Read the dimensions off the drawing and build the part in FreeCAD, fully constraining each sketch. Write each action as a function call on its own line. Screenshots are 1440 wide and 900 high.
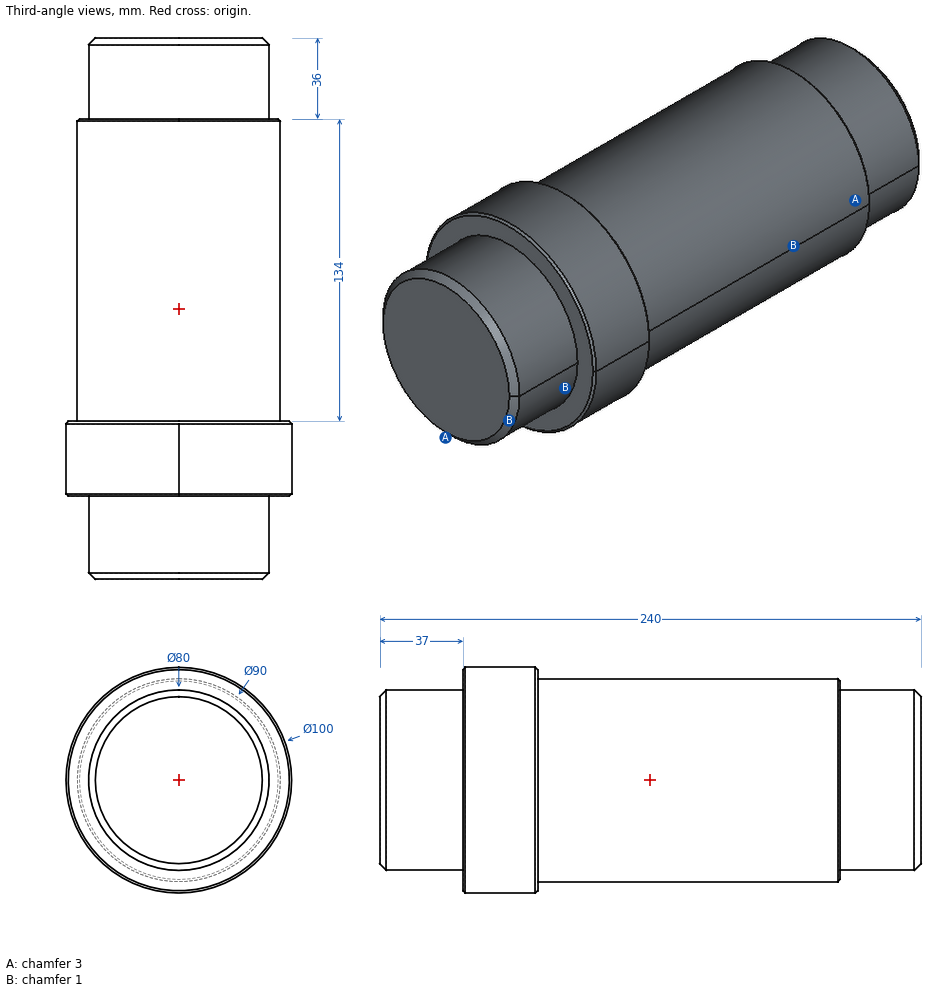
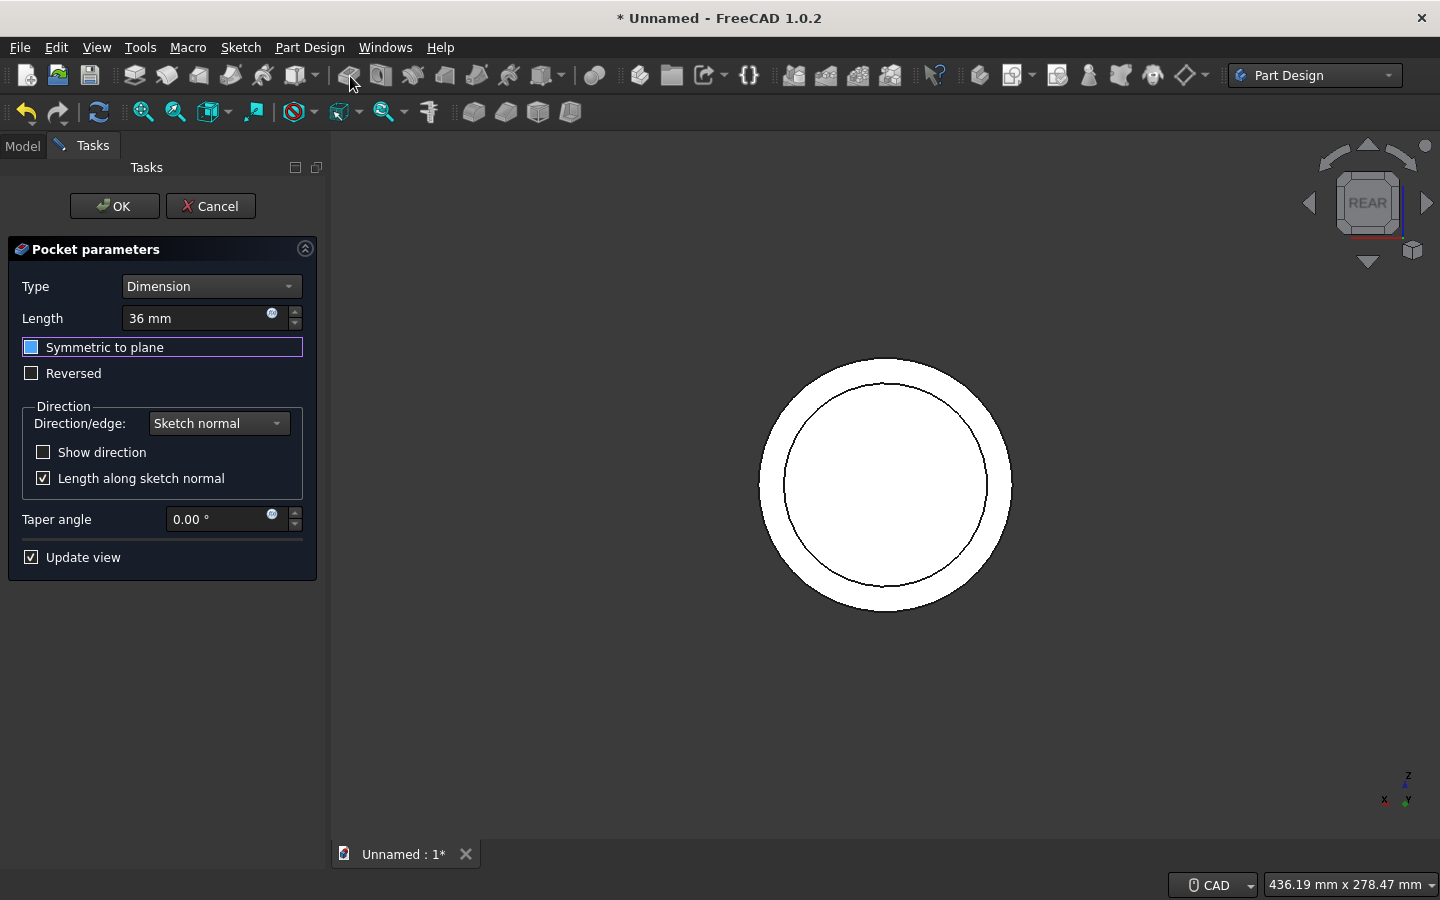
click(115, 206)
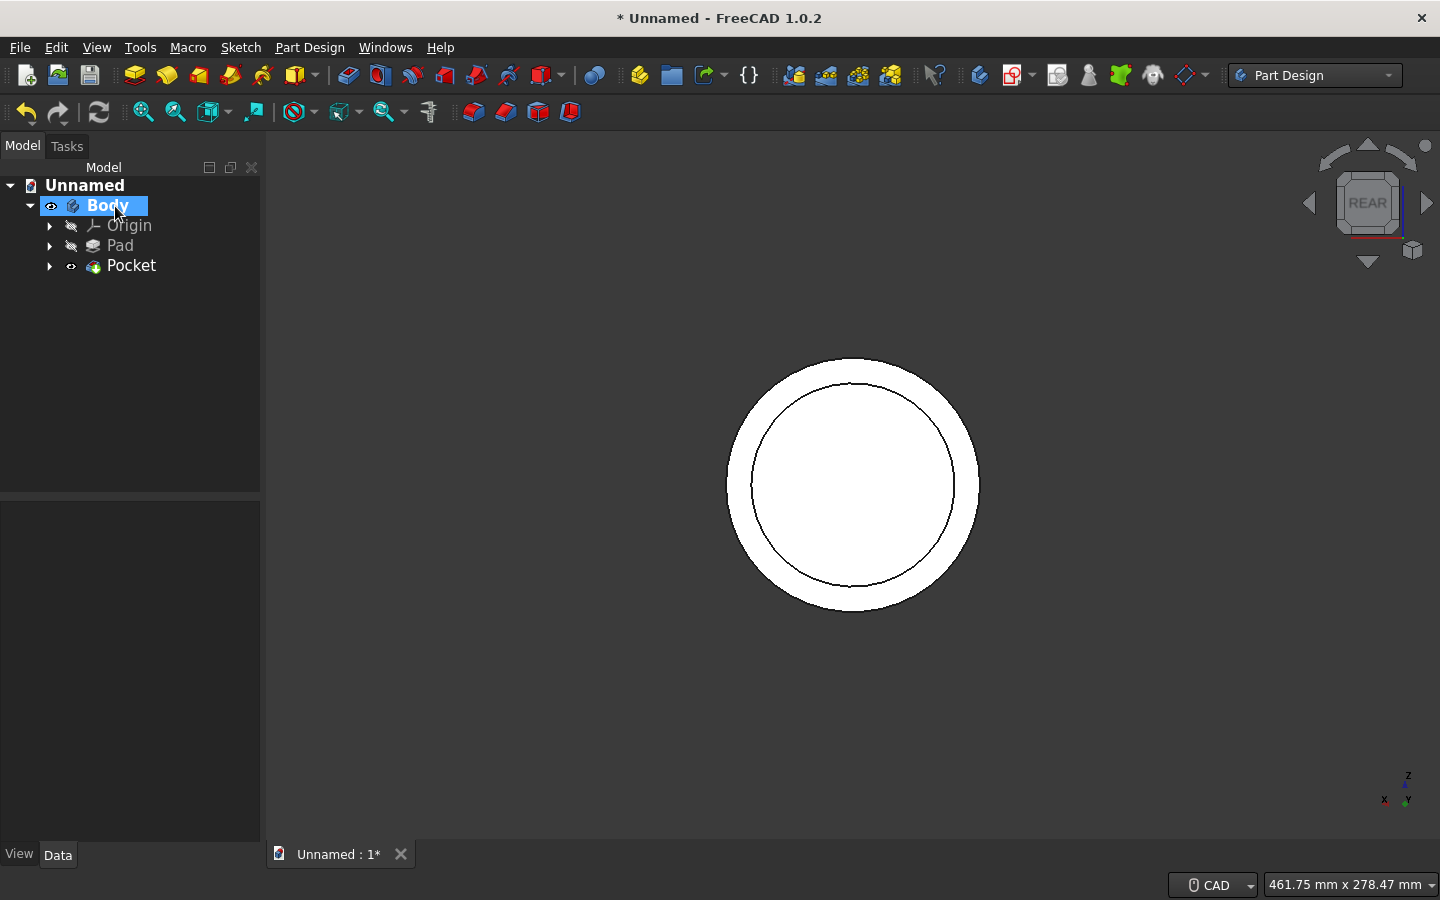
click(144, 112)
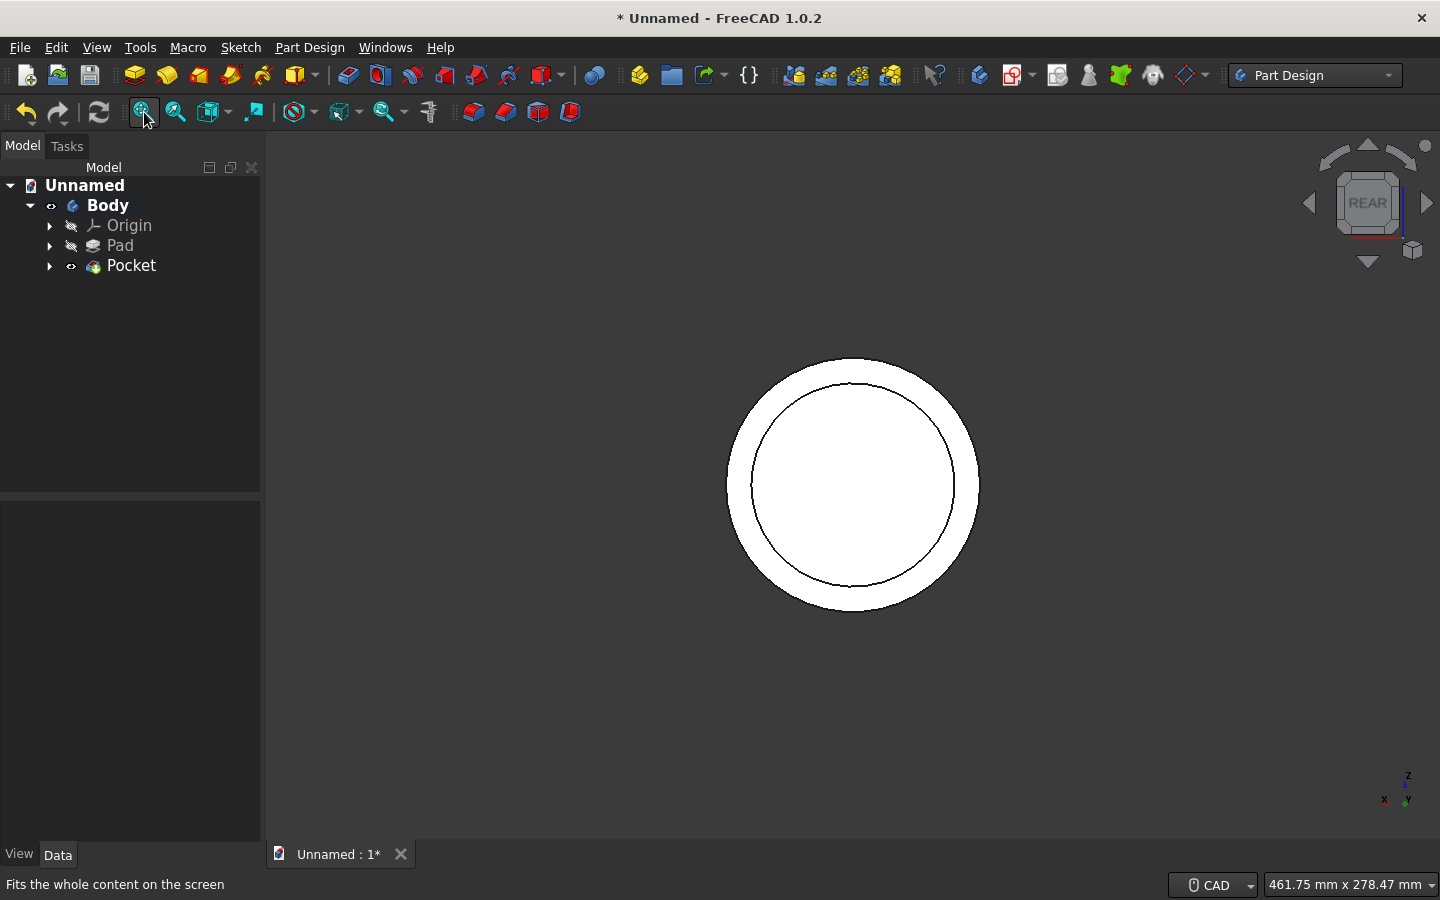
click(50, 226)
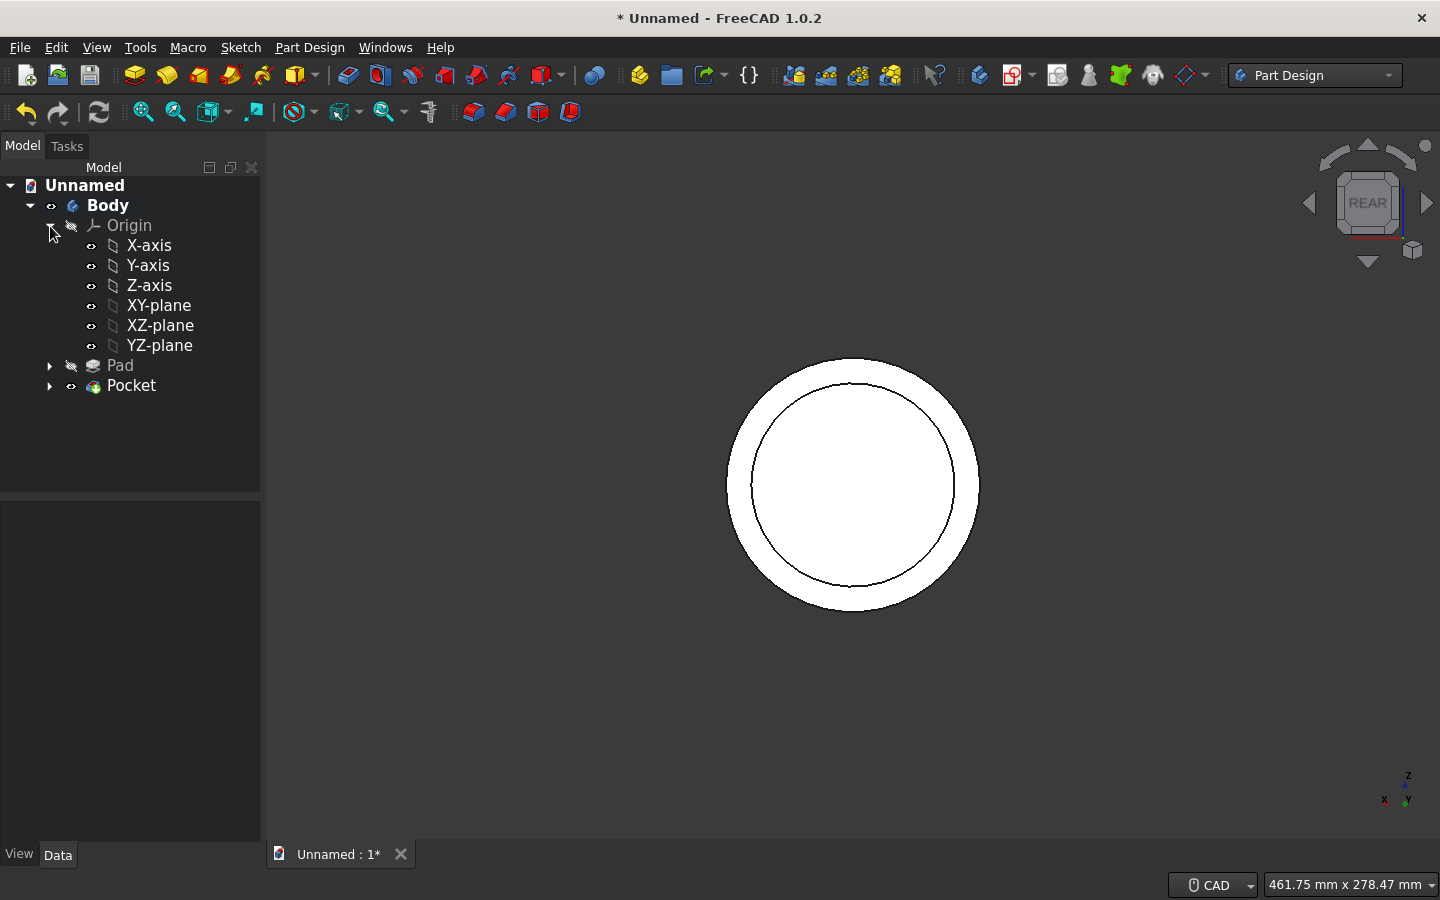
click(136, 326)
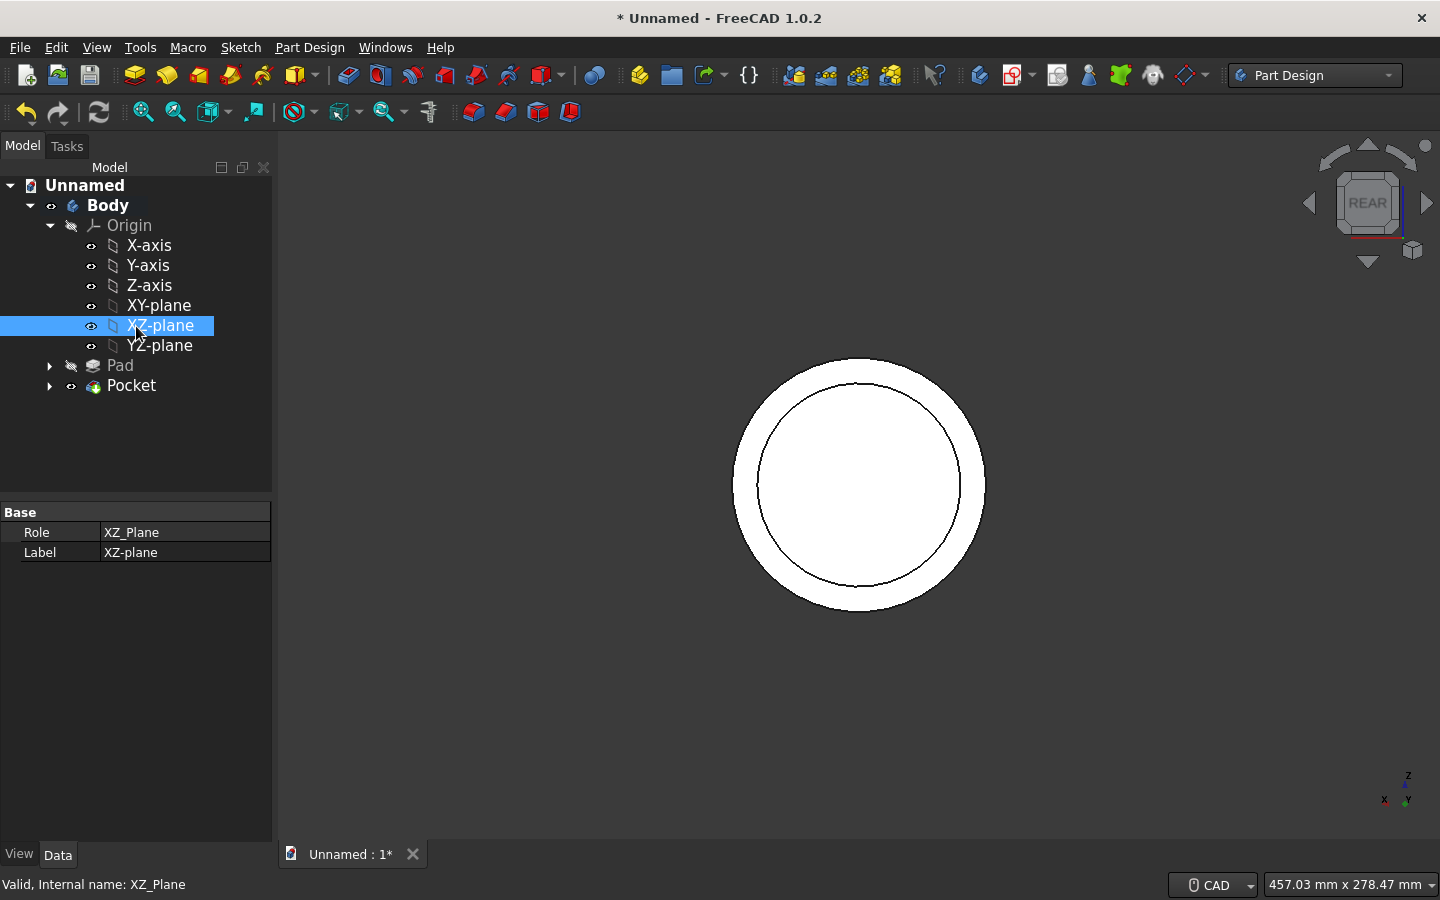
click(1186, 76)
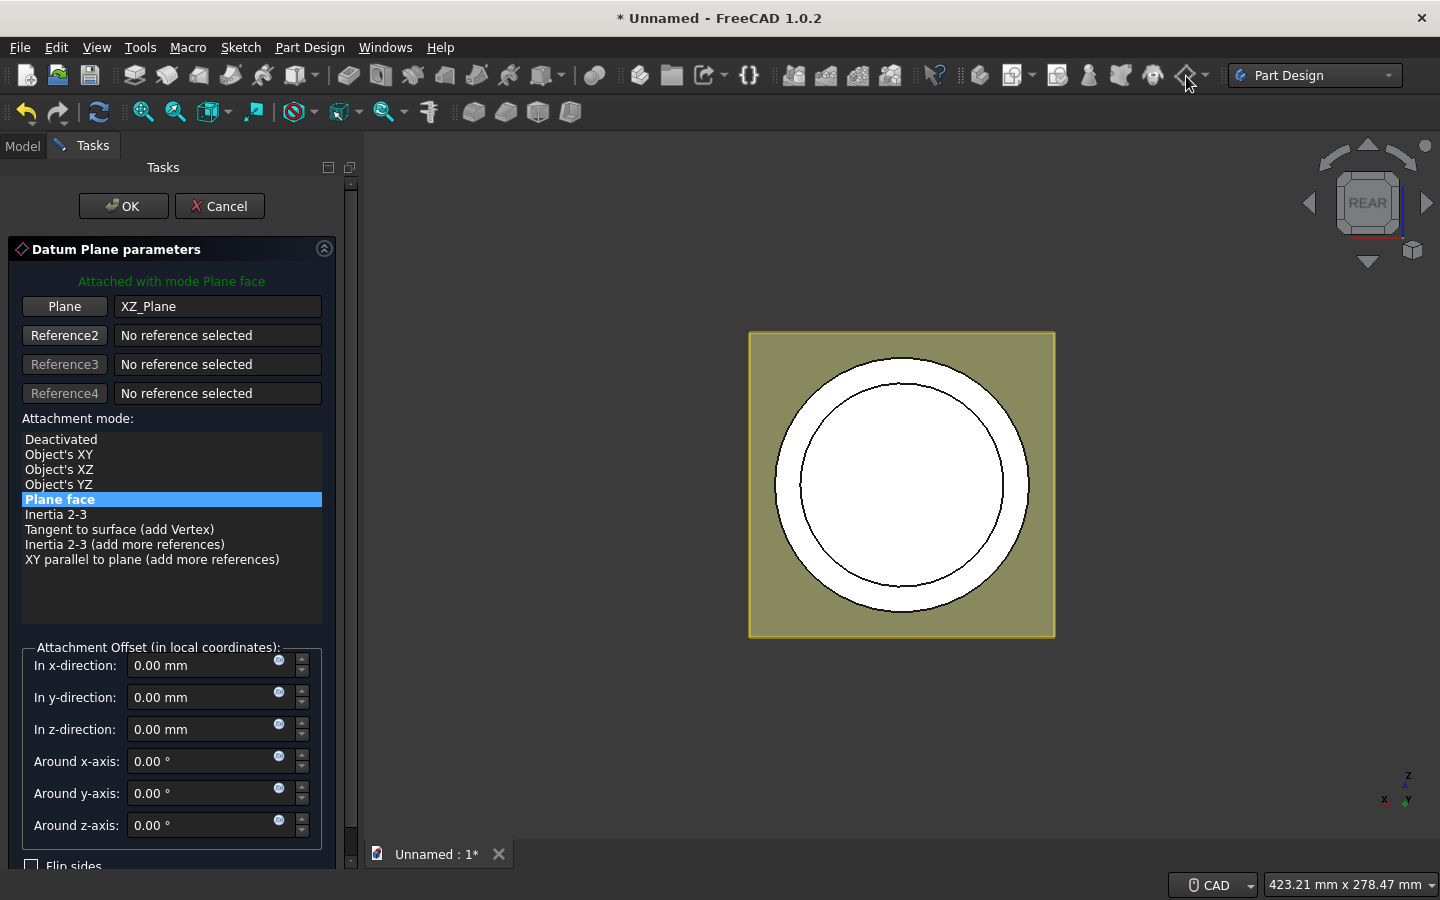
triple_click(210, 729)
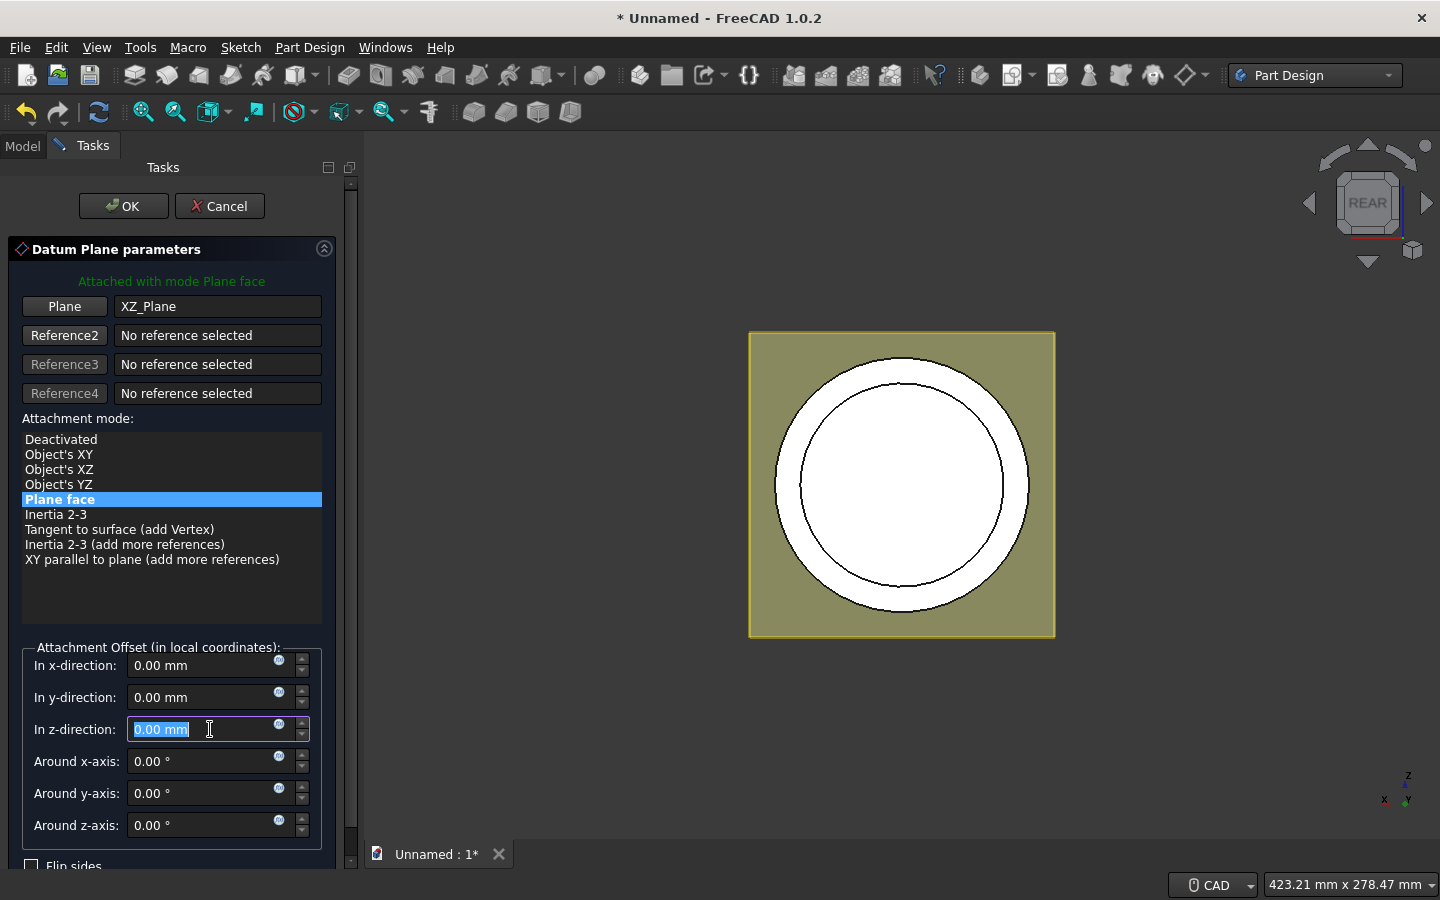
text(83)
key(Tab)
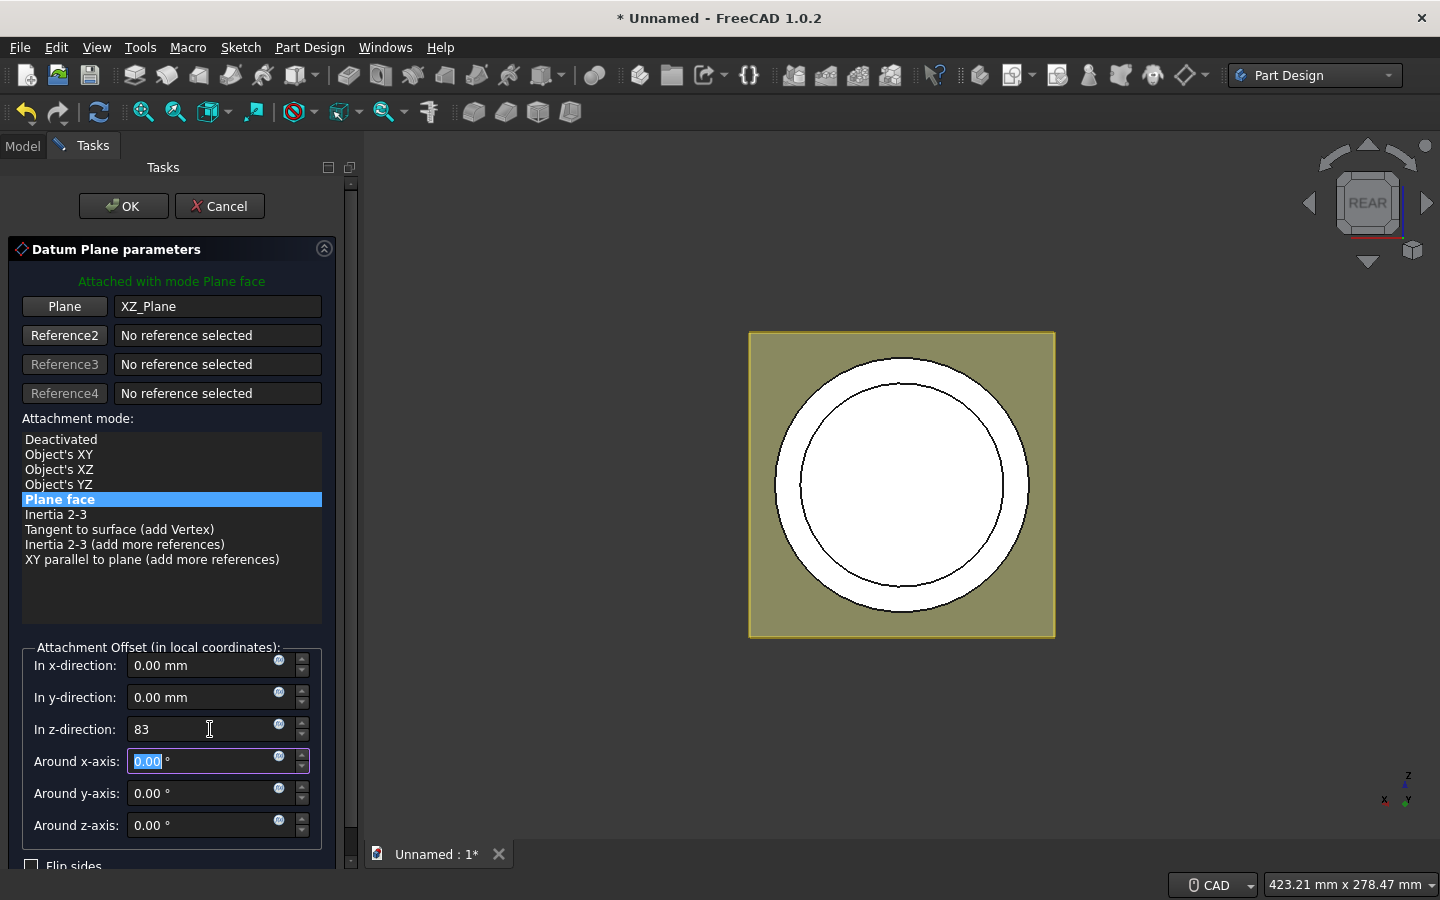
click(124, 206)